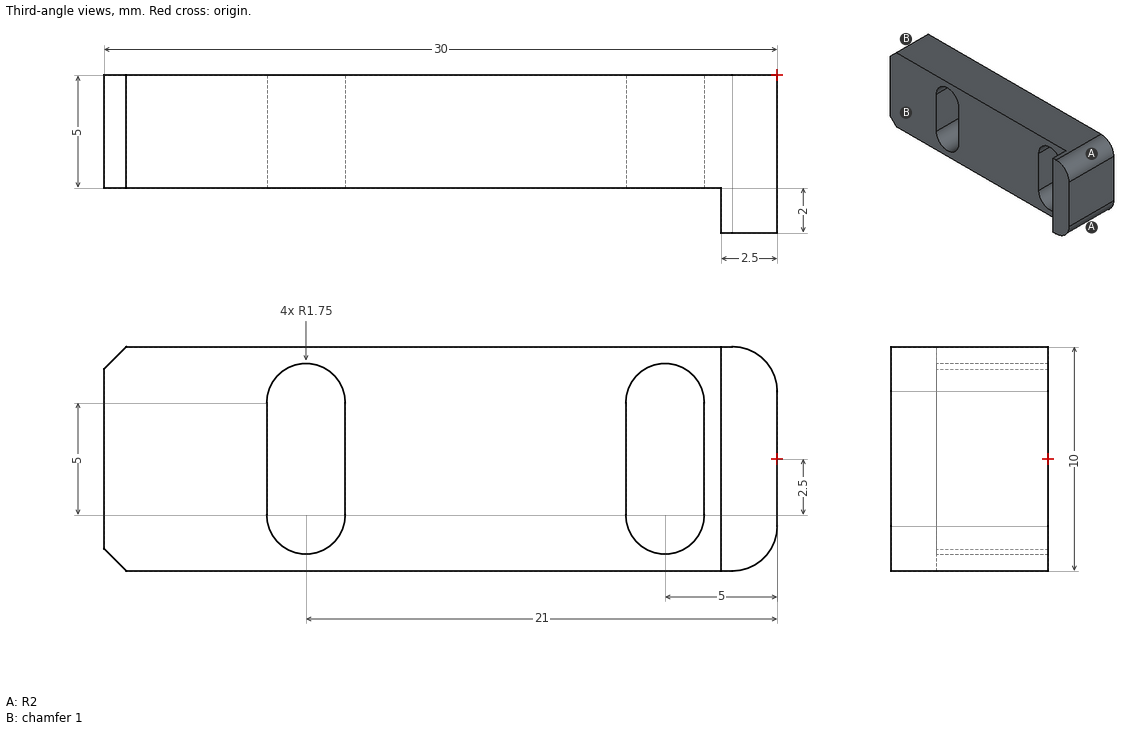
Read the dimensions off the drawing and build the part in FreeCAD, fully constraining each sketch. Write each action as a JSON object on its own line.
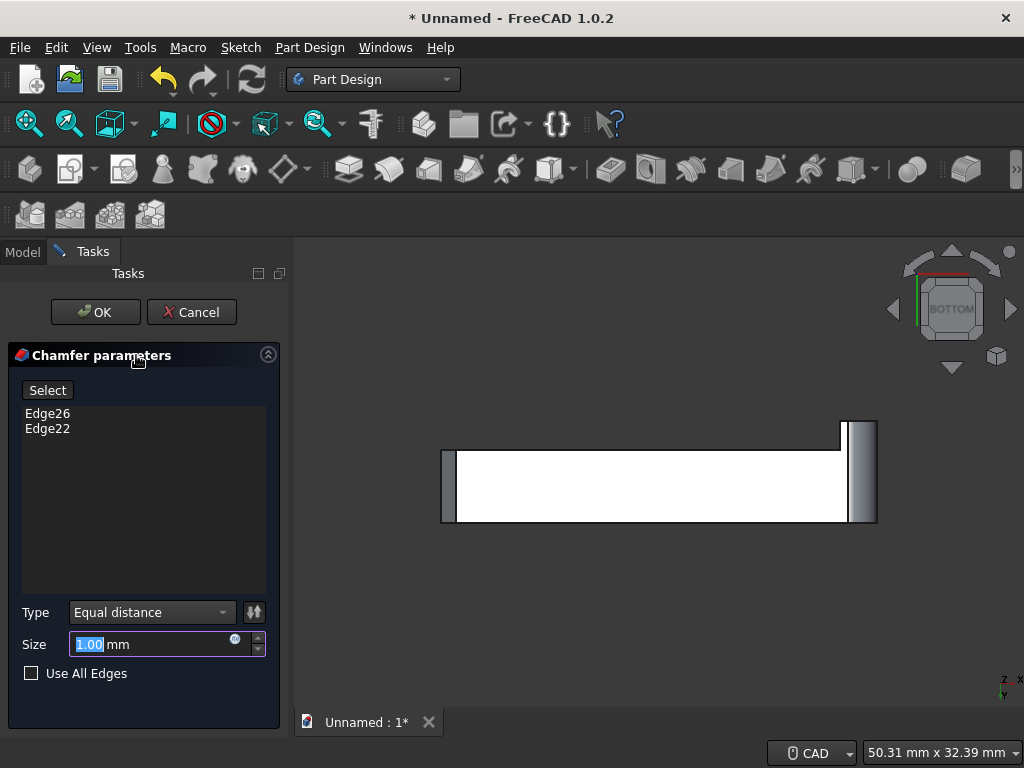
{"action": "type", "text": "1"}
{"action": "key", "text": "Tab"}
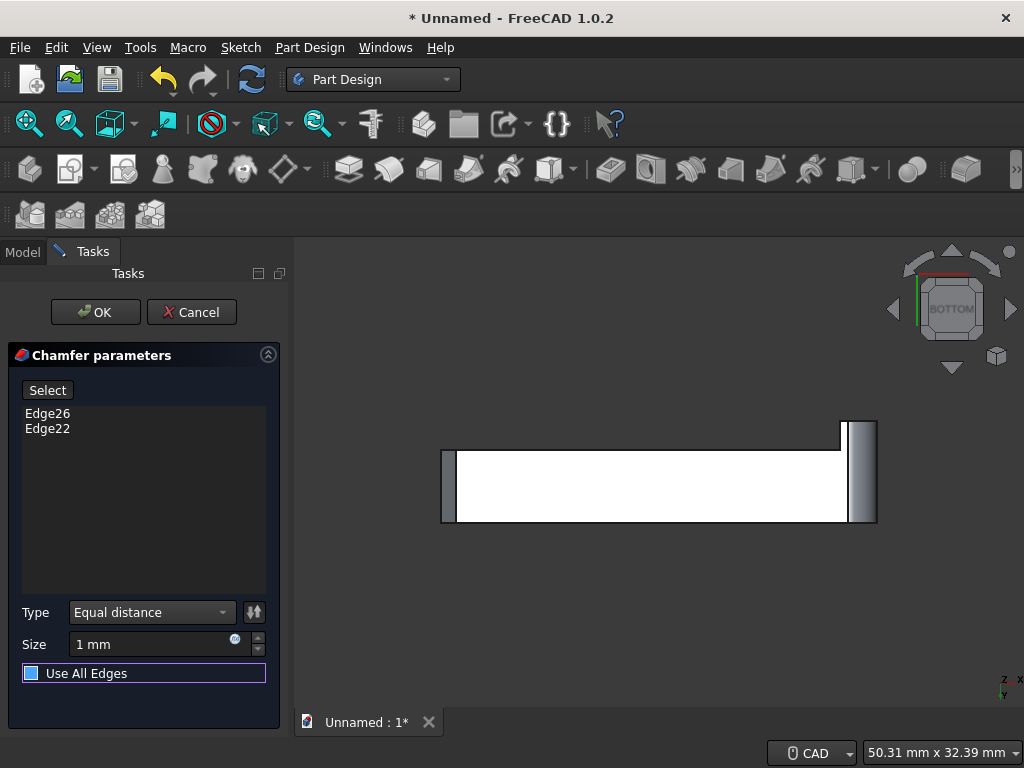
{"action": "left_click", "coordinate": [96, 312]}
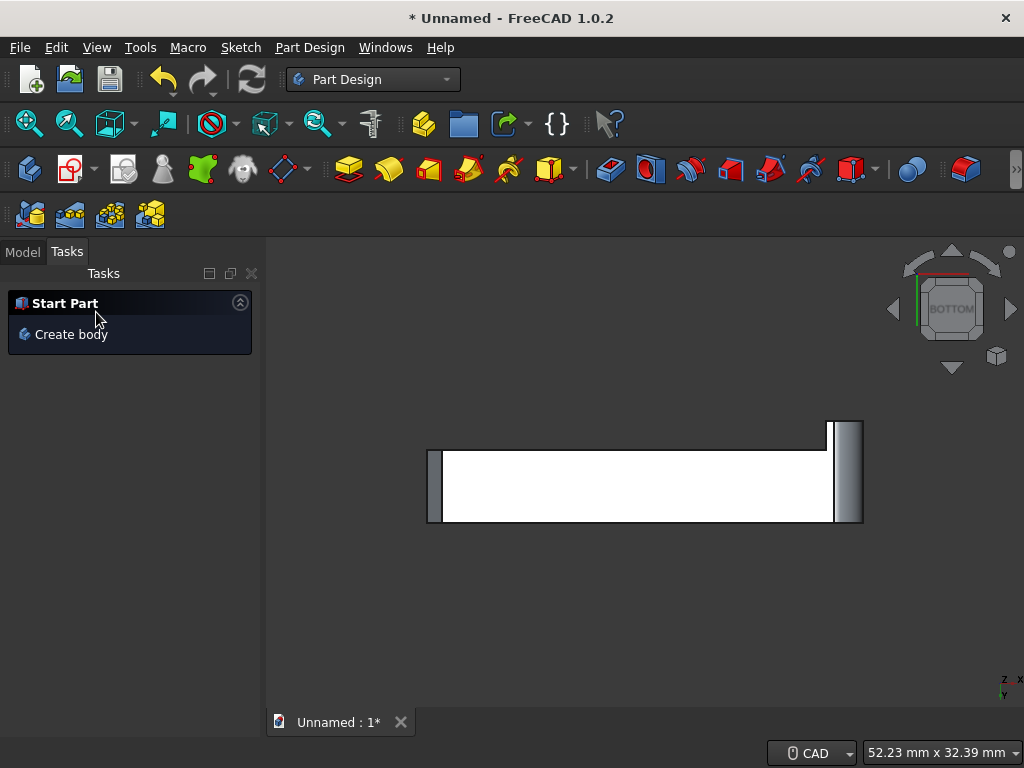
{"action": "key", "text": "0"}